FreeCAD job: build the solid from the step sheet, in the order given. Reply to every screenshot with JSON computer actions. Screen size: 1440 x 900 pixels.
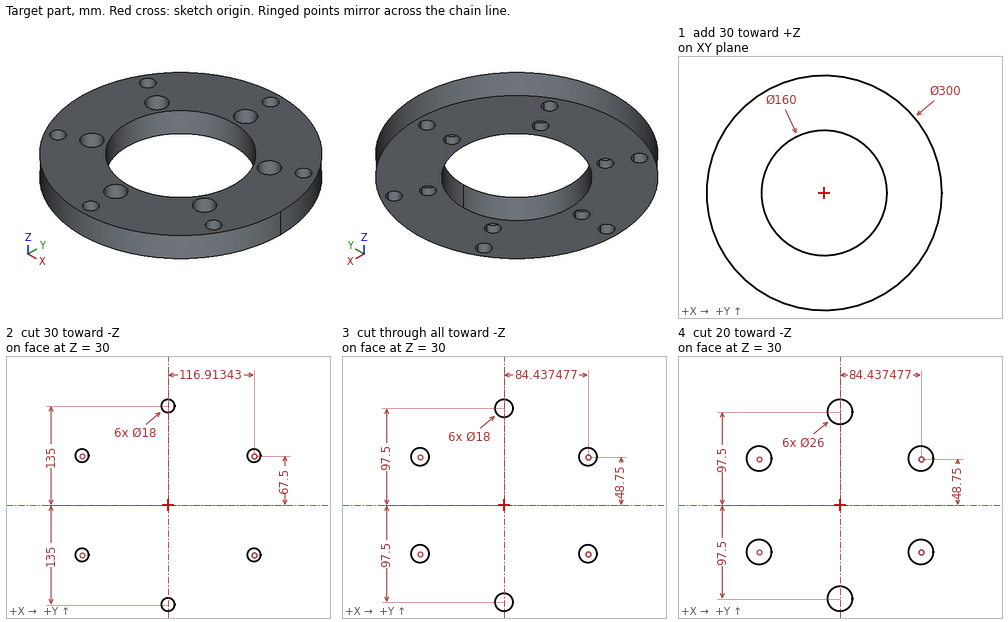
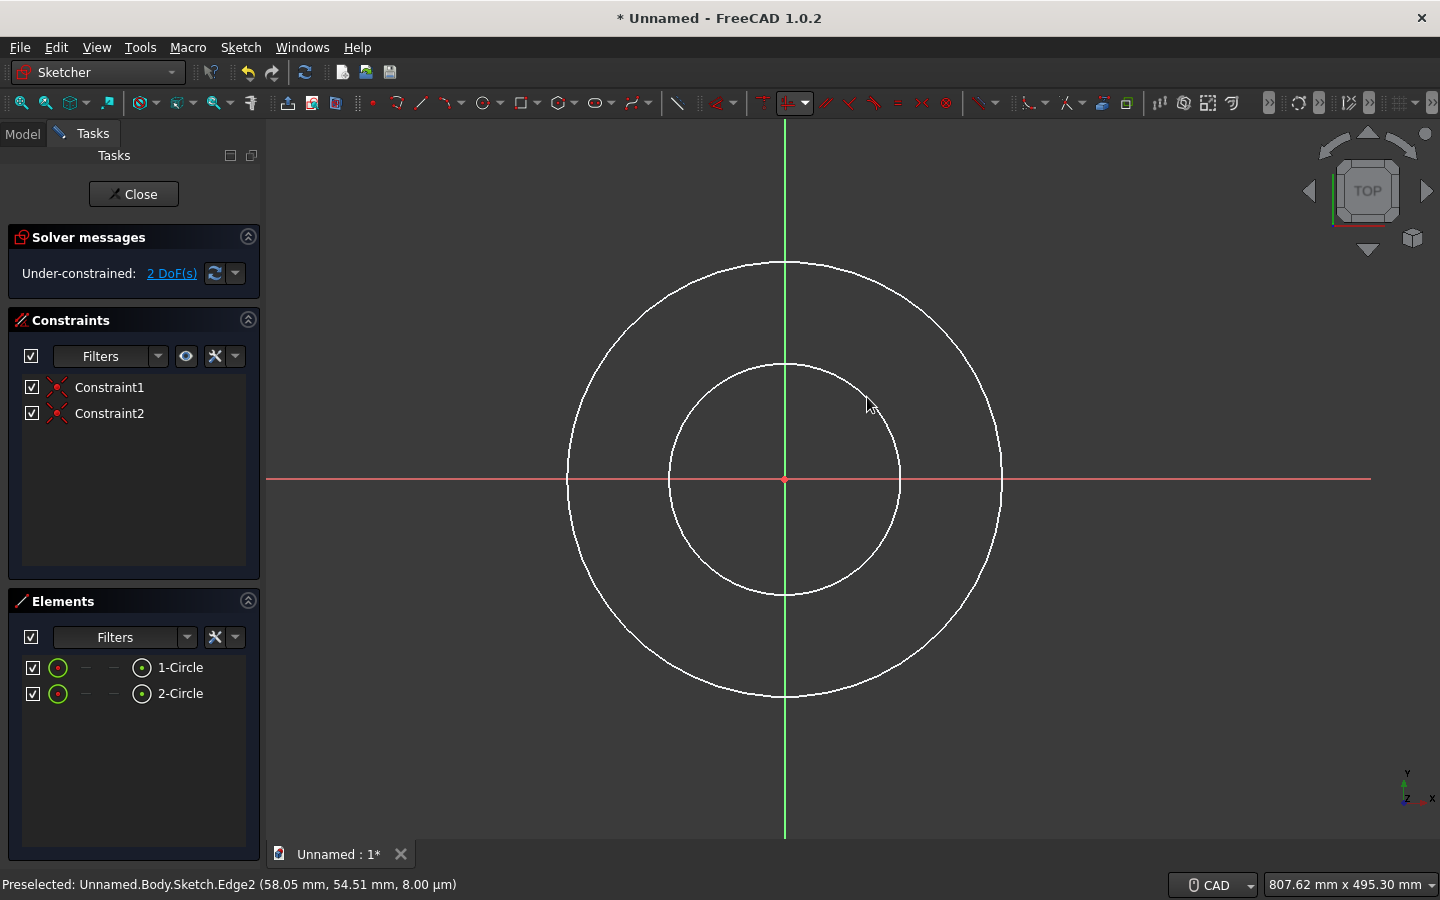
{"action": "left_click", "coordinate": [938, 325]}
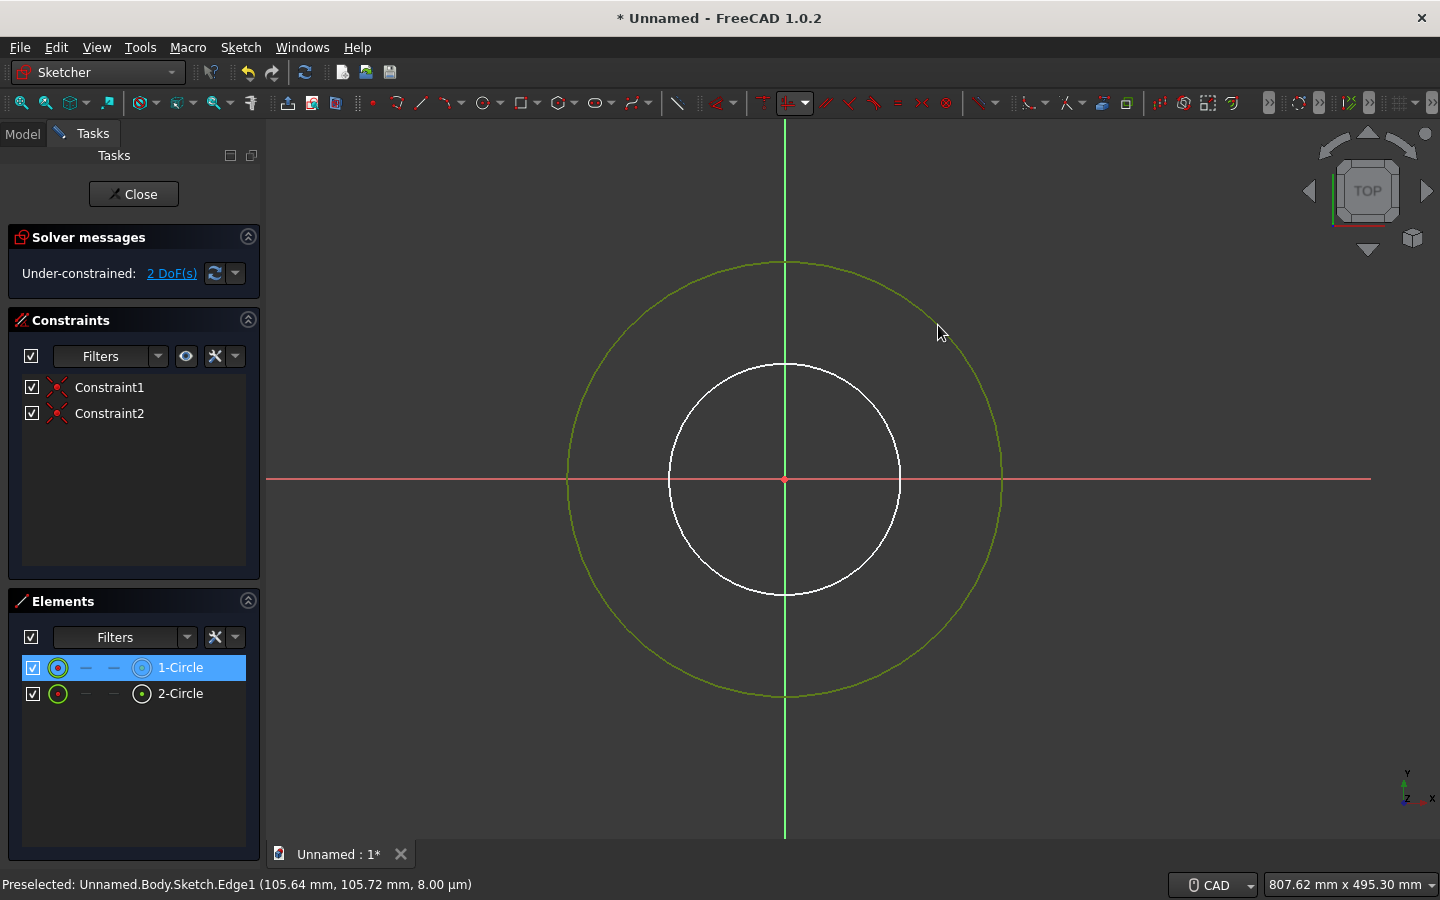
{"action": "key", "text": "k o"}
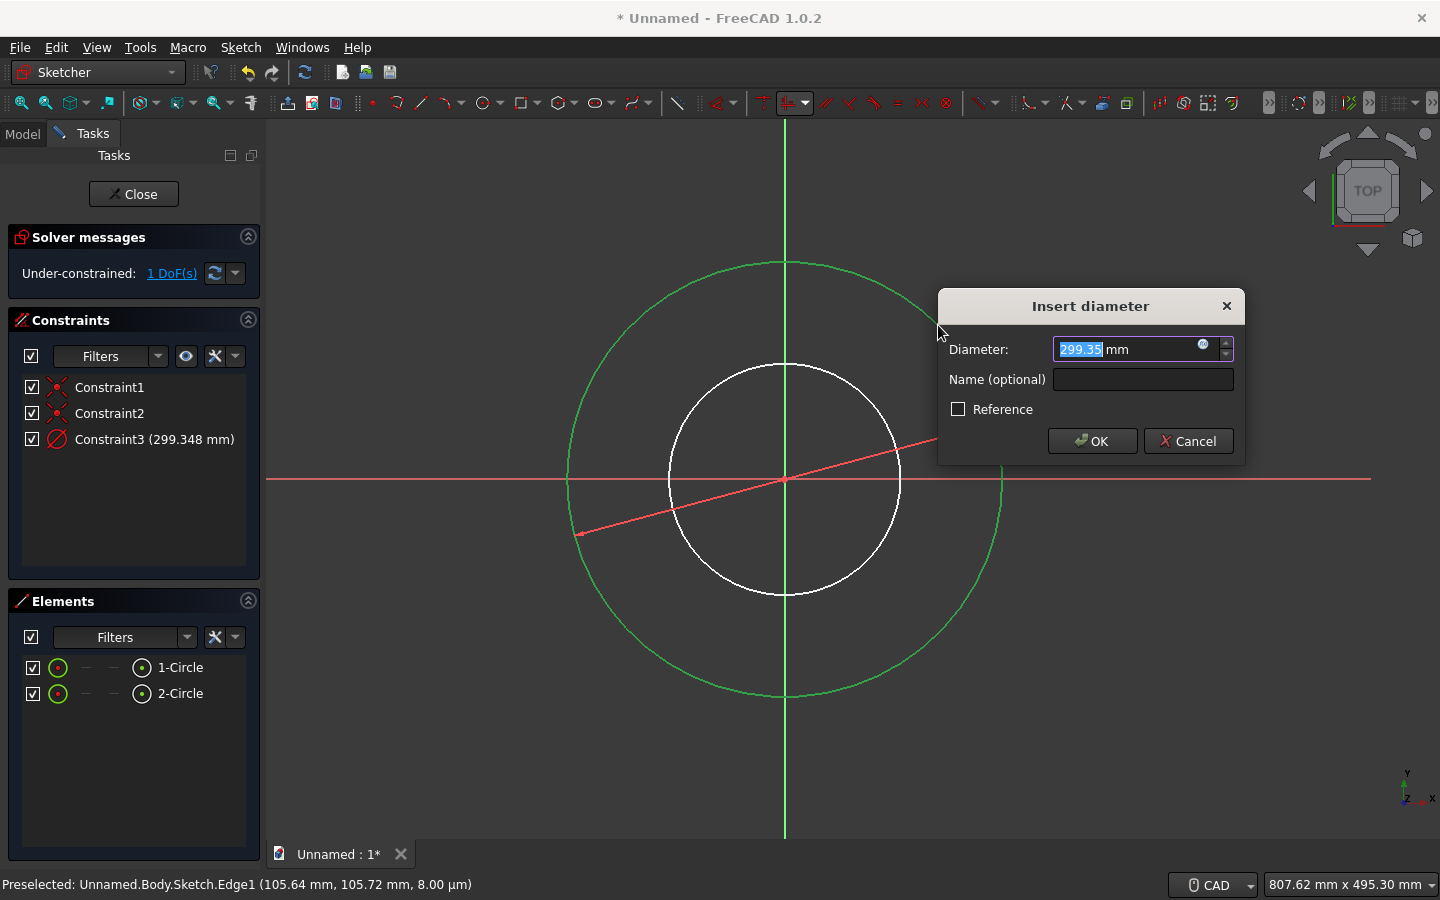
{"action": "type", "text": "300"}
{"action": "key", "text": "Return"}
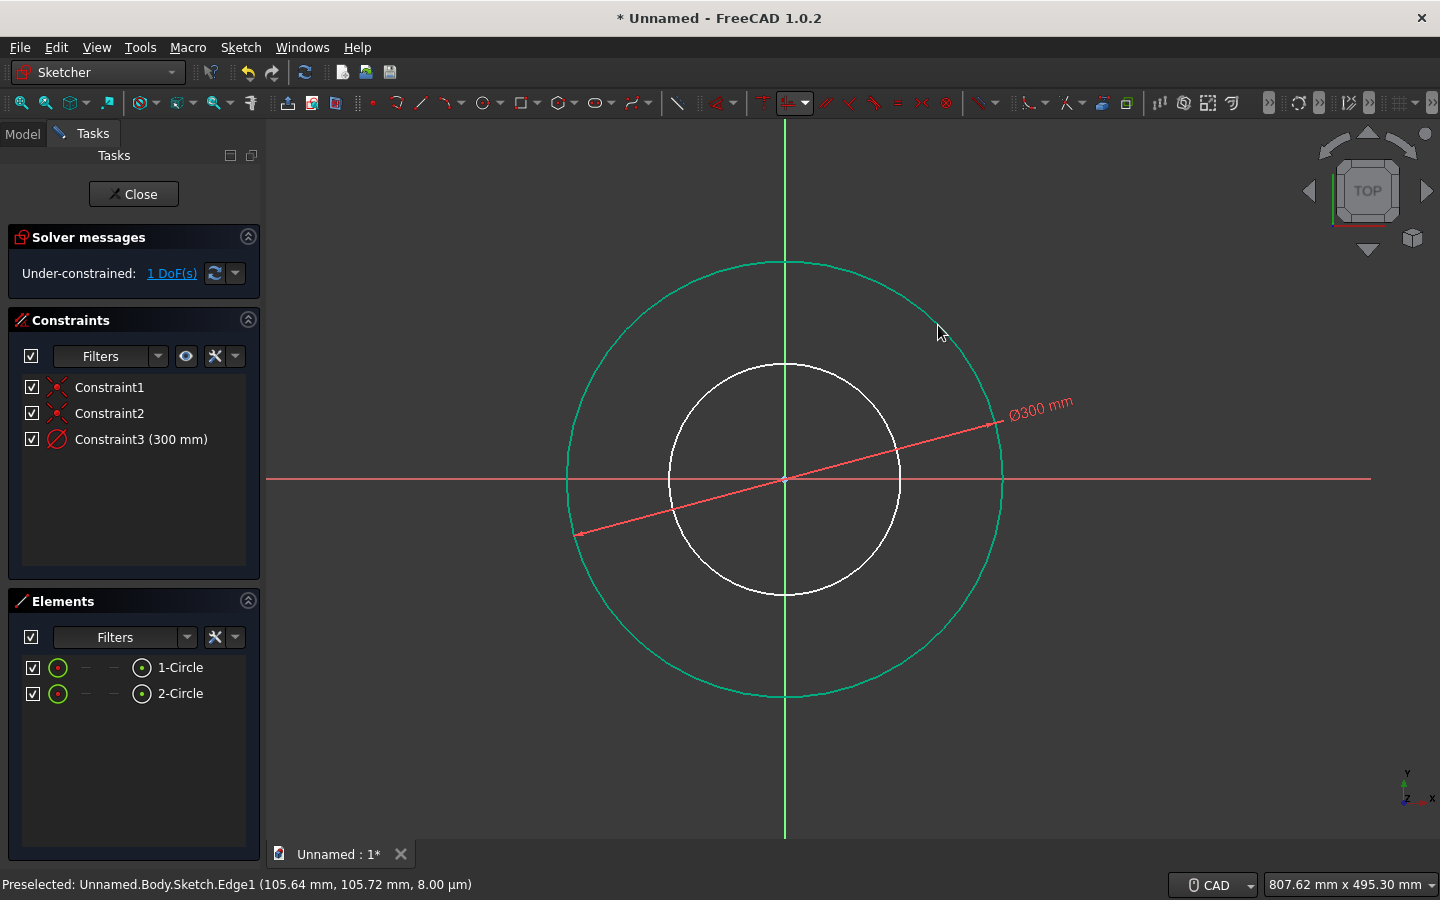
{"action": "left_click", "coordinate": [866, 397]}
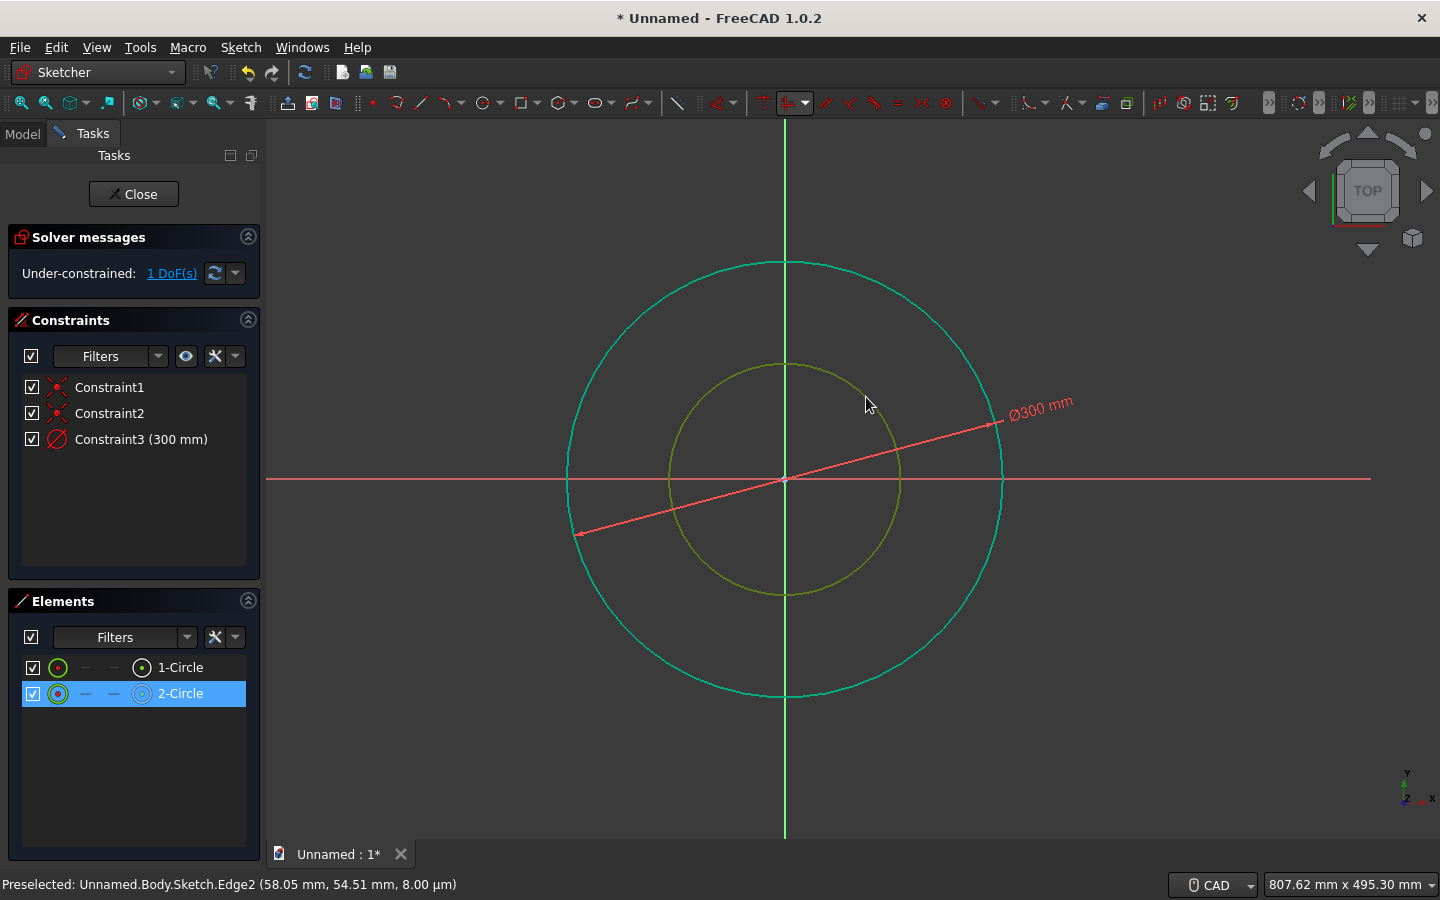
{"action": "key", "text": "k o"}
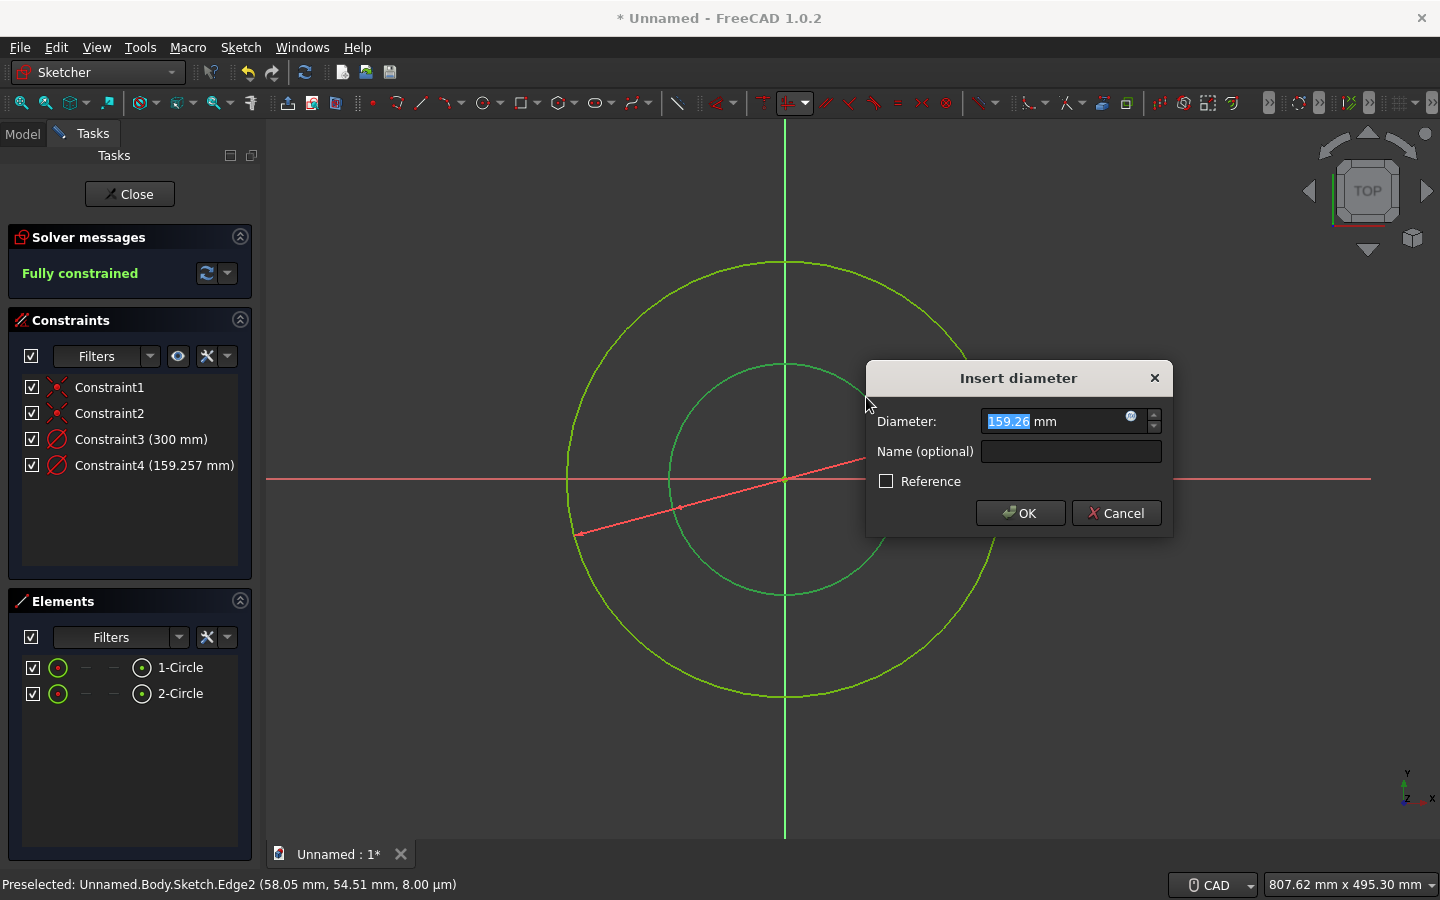
{"action": "type", "text": "160"}
{"action": "key", "text": "Return"}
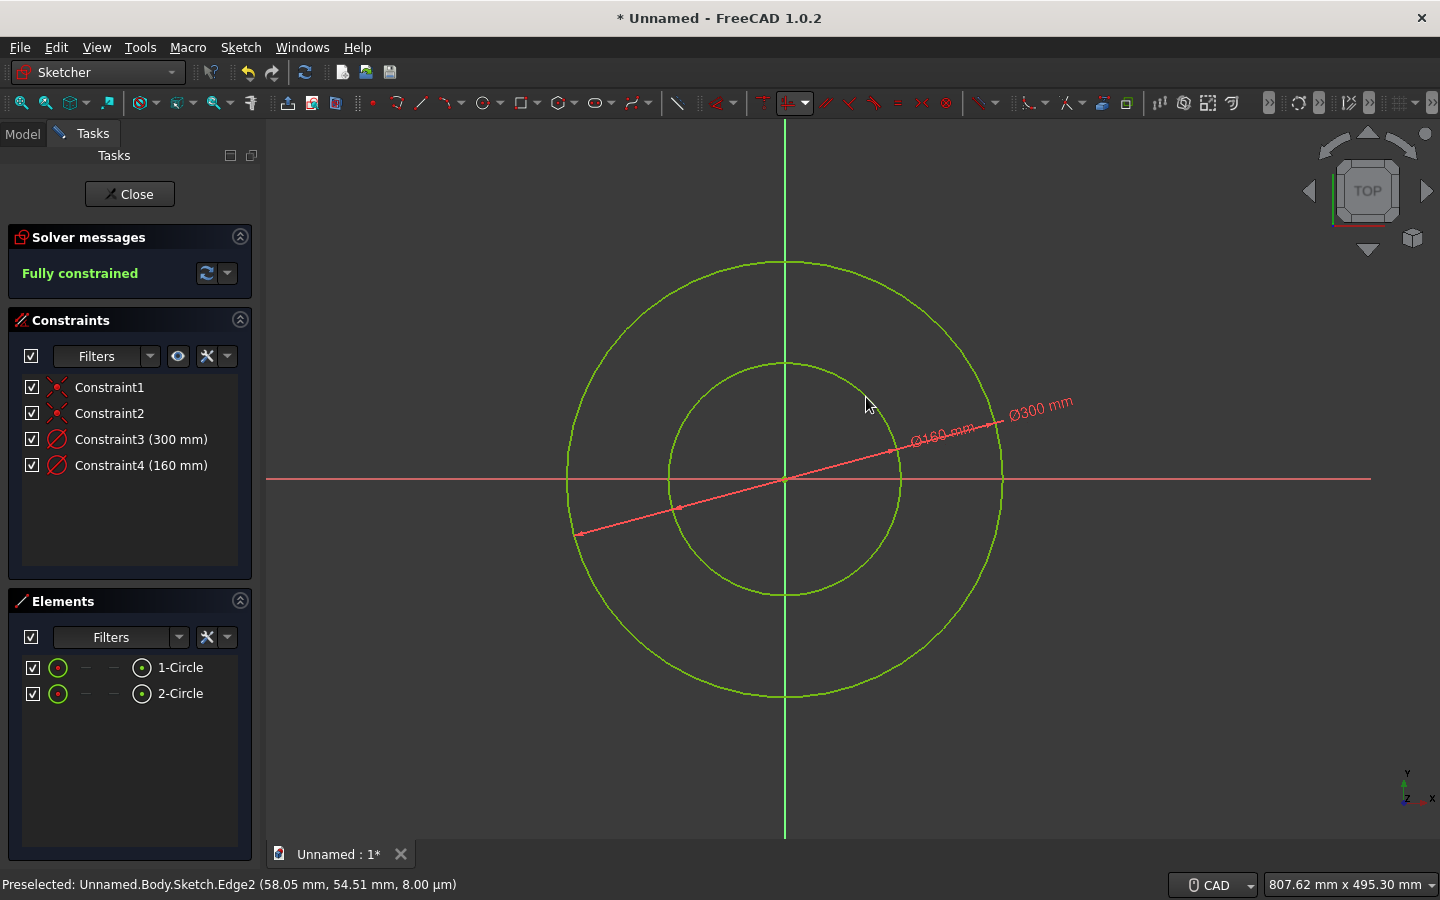
{"action": "left_click", "coordinate": [130, 194]}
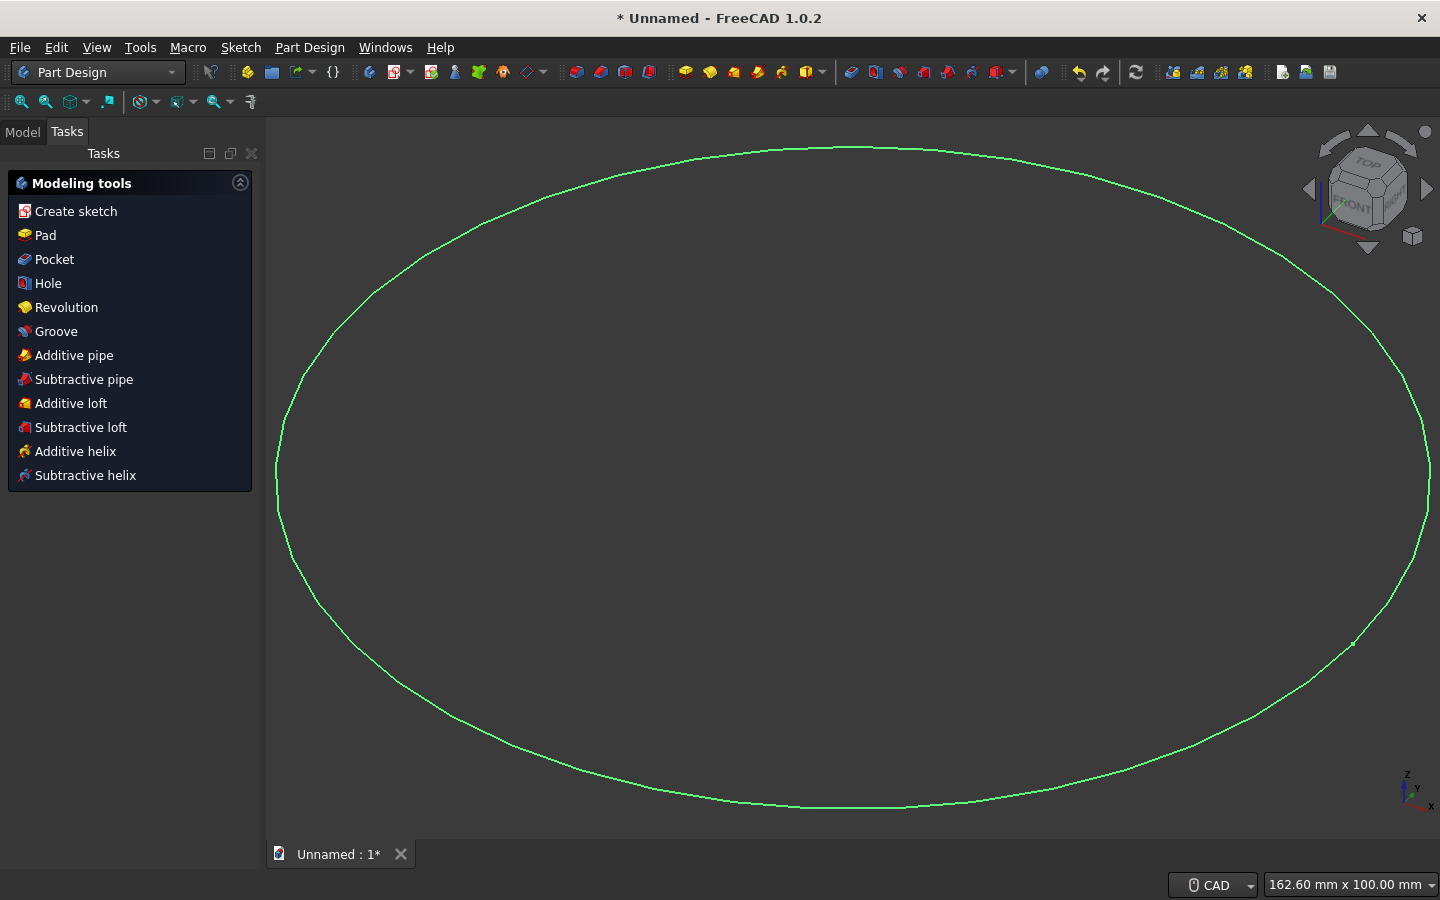
{"action": "left_click", "coordinate": [686, 72]}